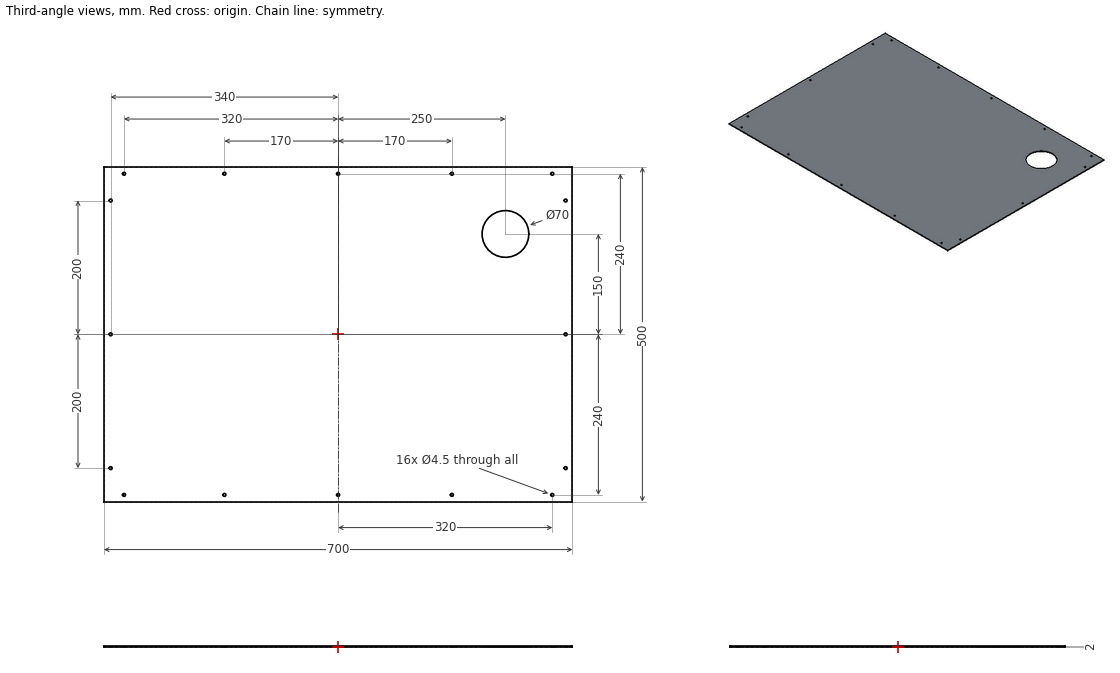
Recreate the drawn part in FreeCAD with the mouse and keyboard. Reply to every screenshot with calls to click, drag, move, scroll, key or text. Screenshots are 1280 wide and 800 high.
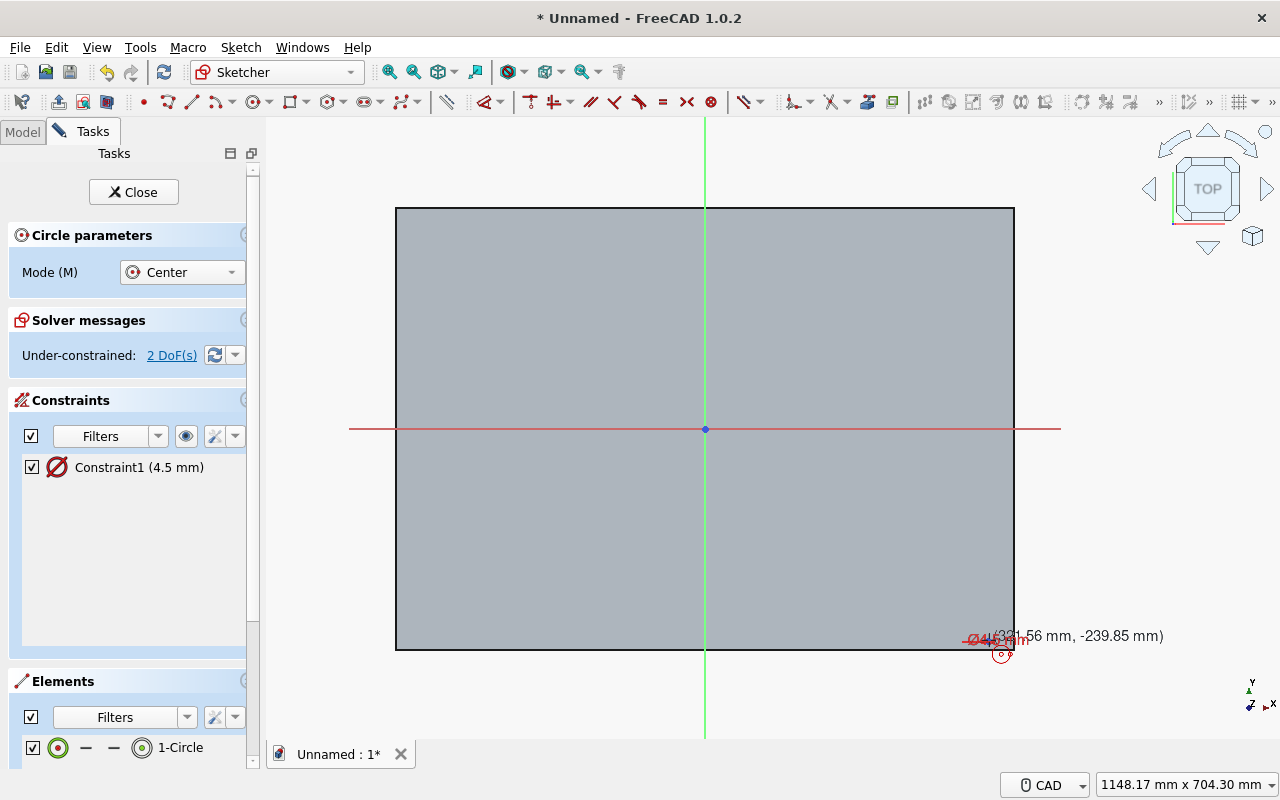
scroll(405, 429, up, 13)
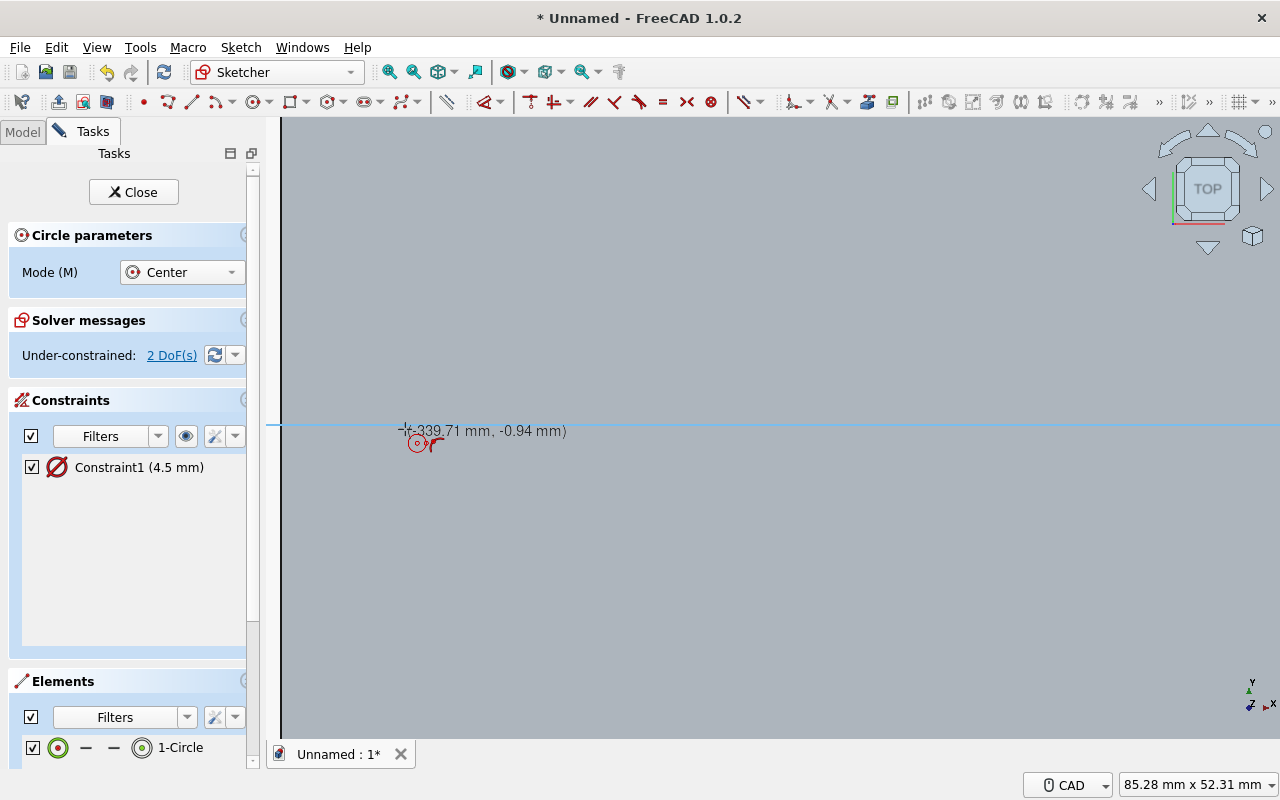
scroll(405, 428, down, 13)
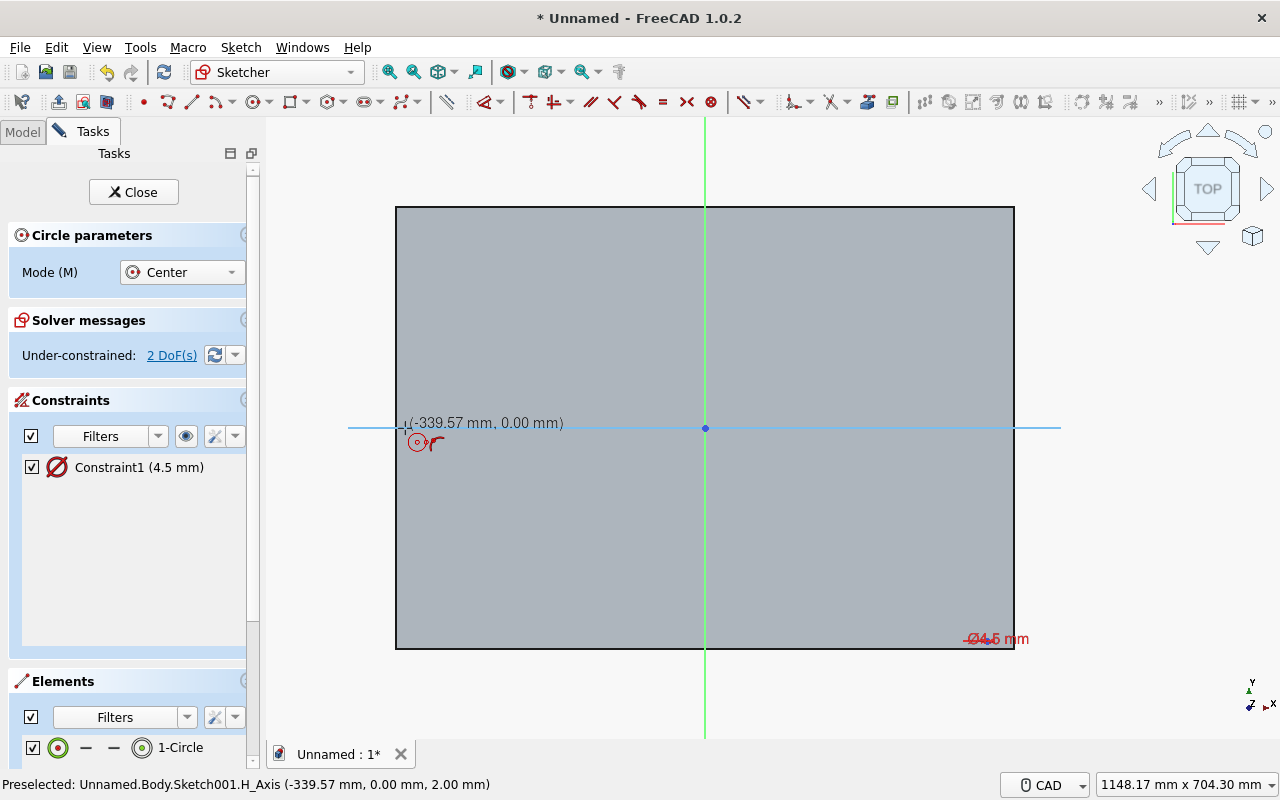
click(405, 428)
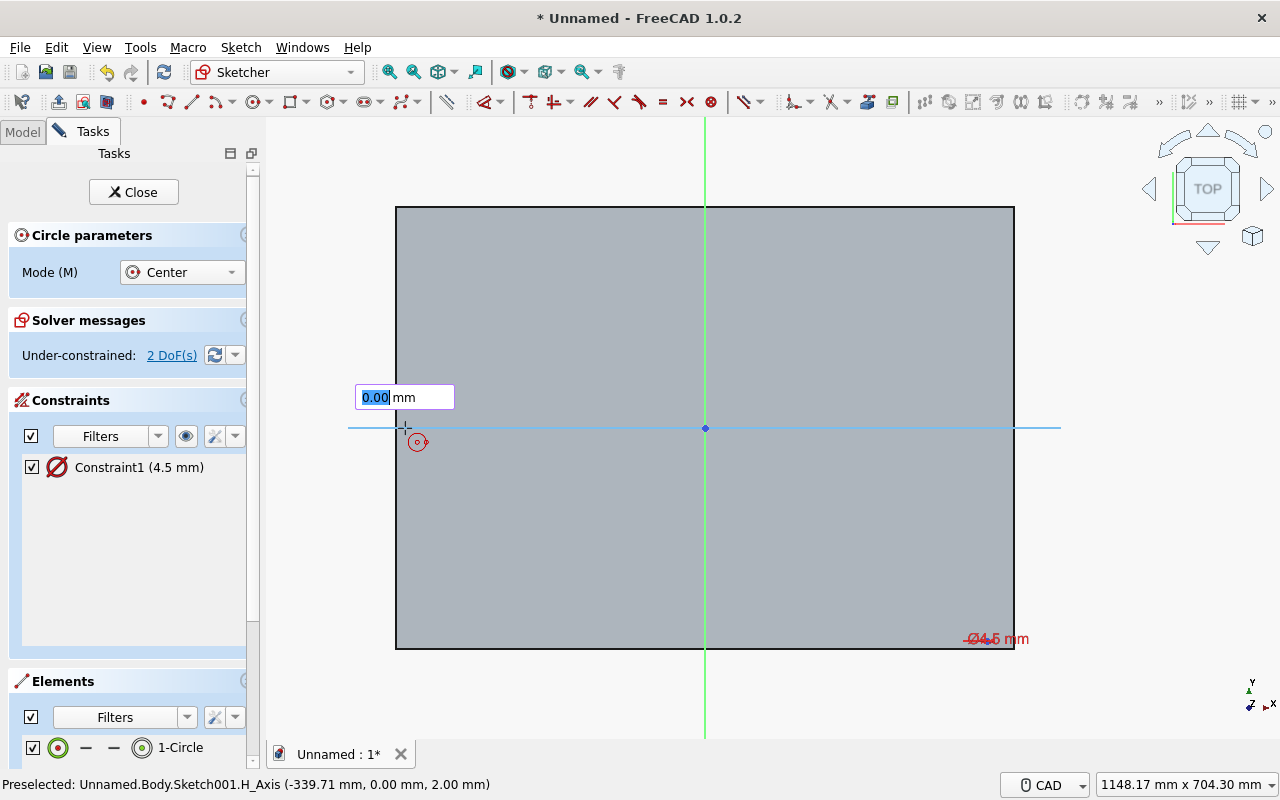
scroll(404, 430, up, 11)
move(404, 427)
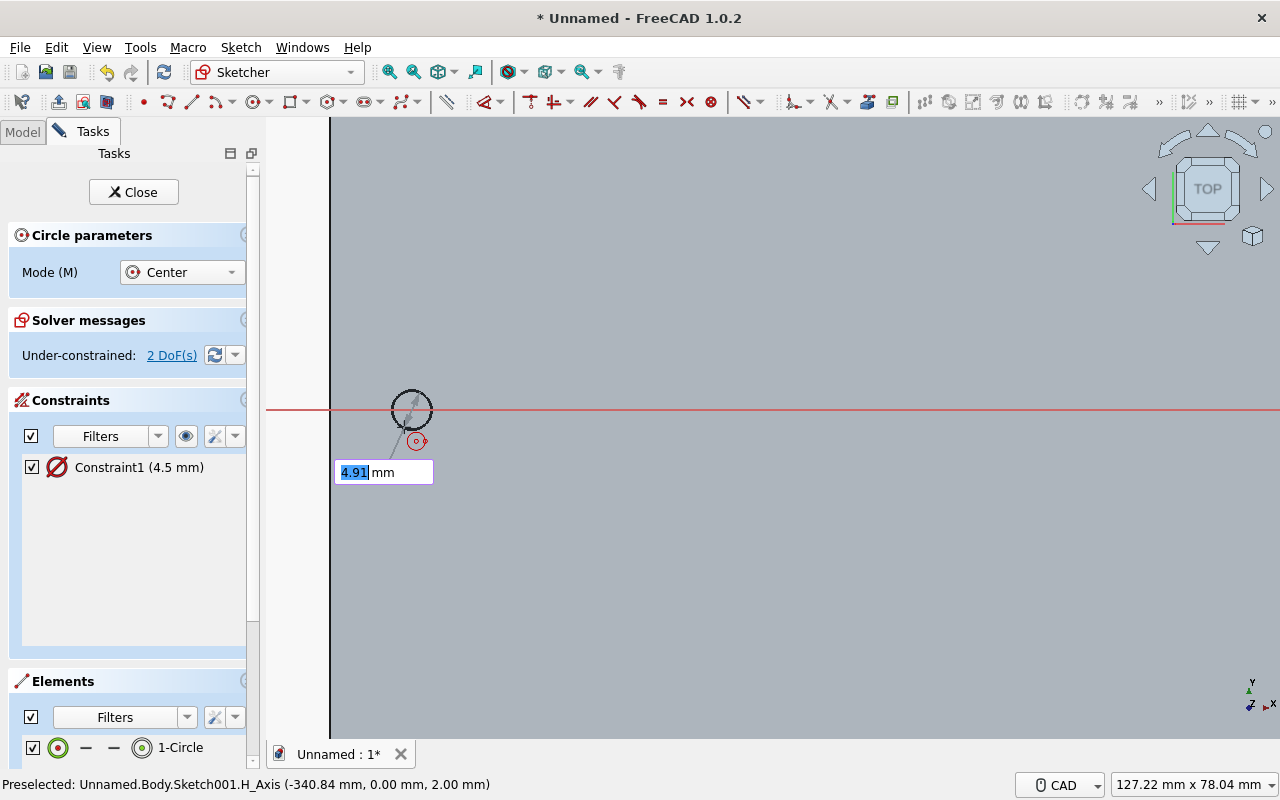
text(4.5)
key(Return)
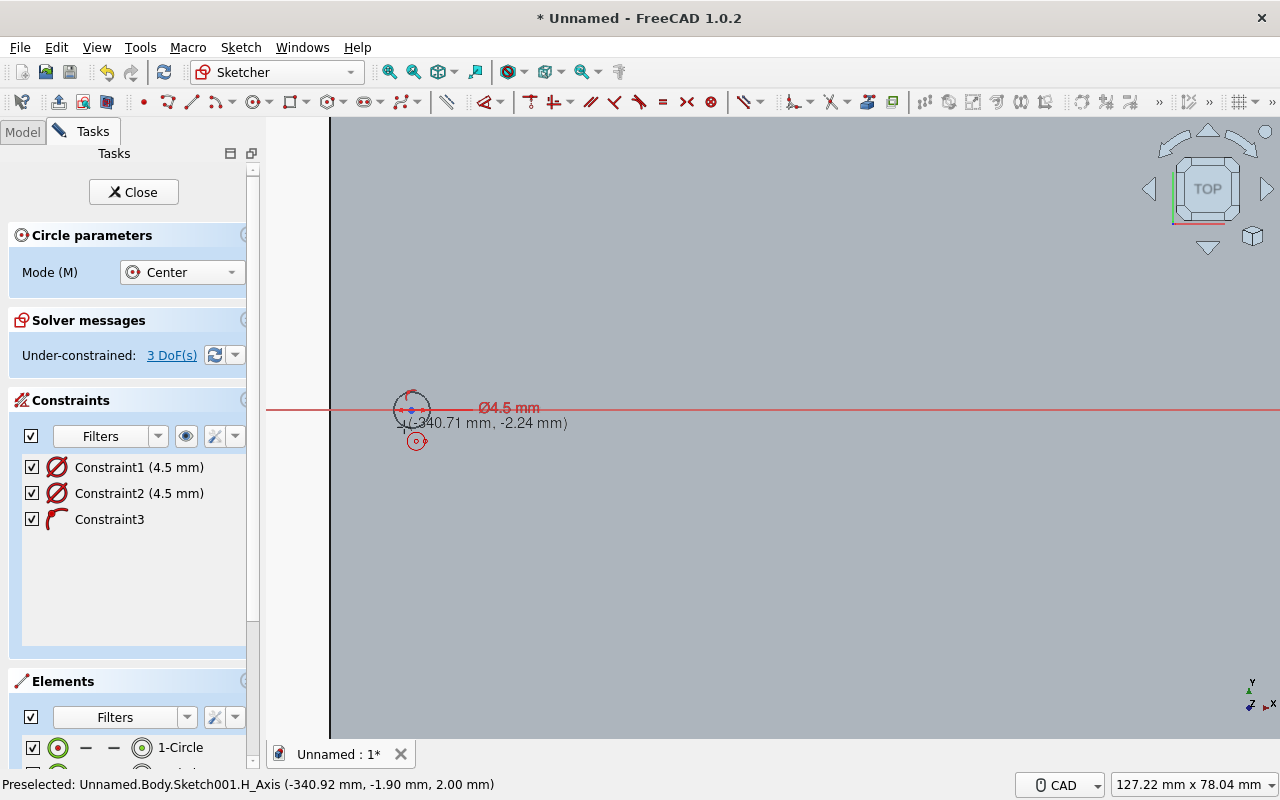
scroll(404, 430, down, 11)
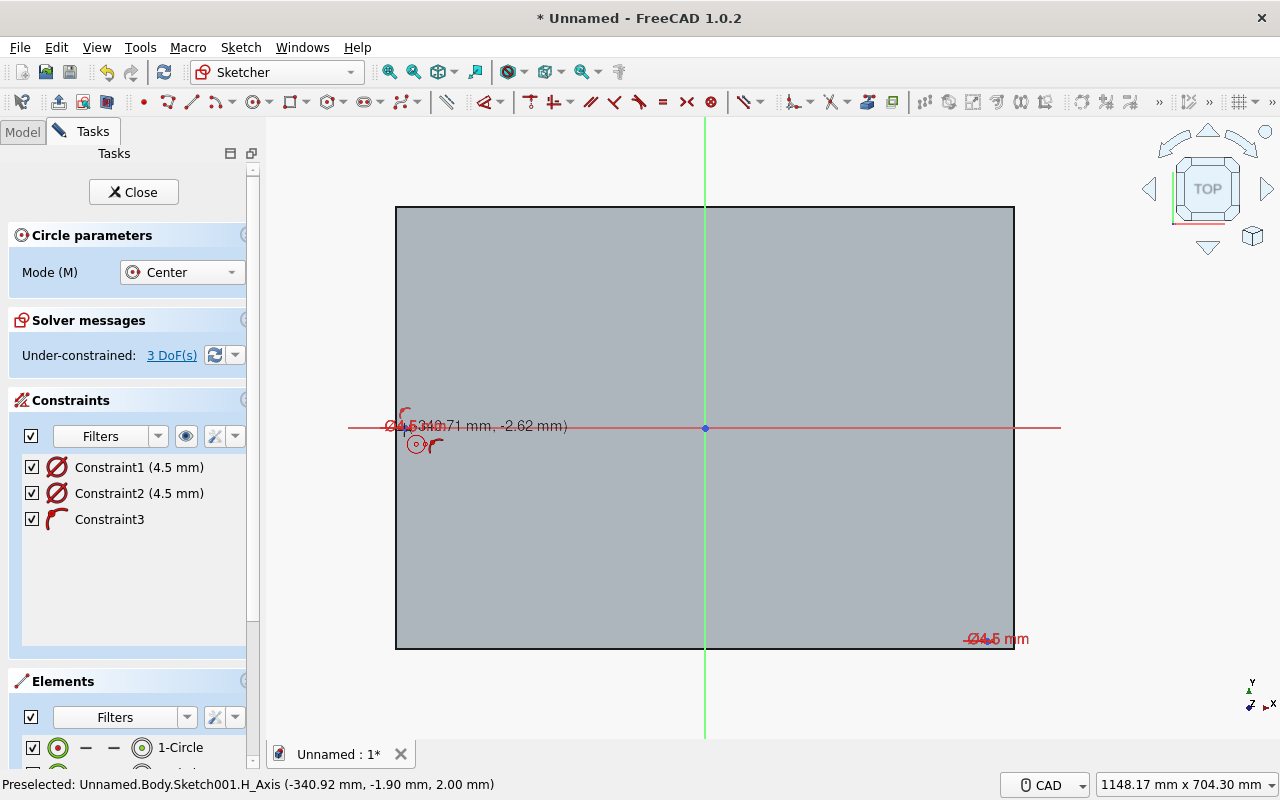
scroll(705, 640, up, 13)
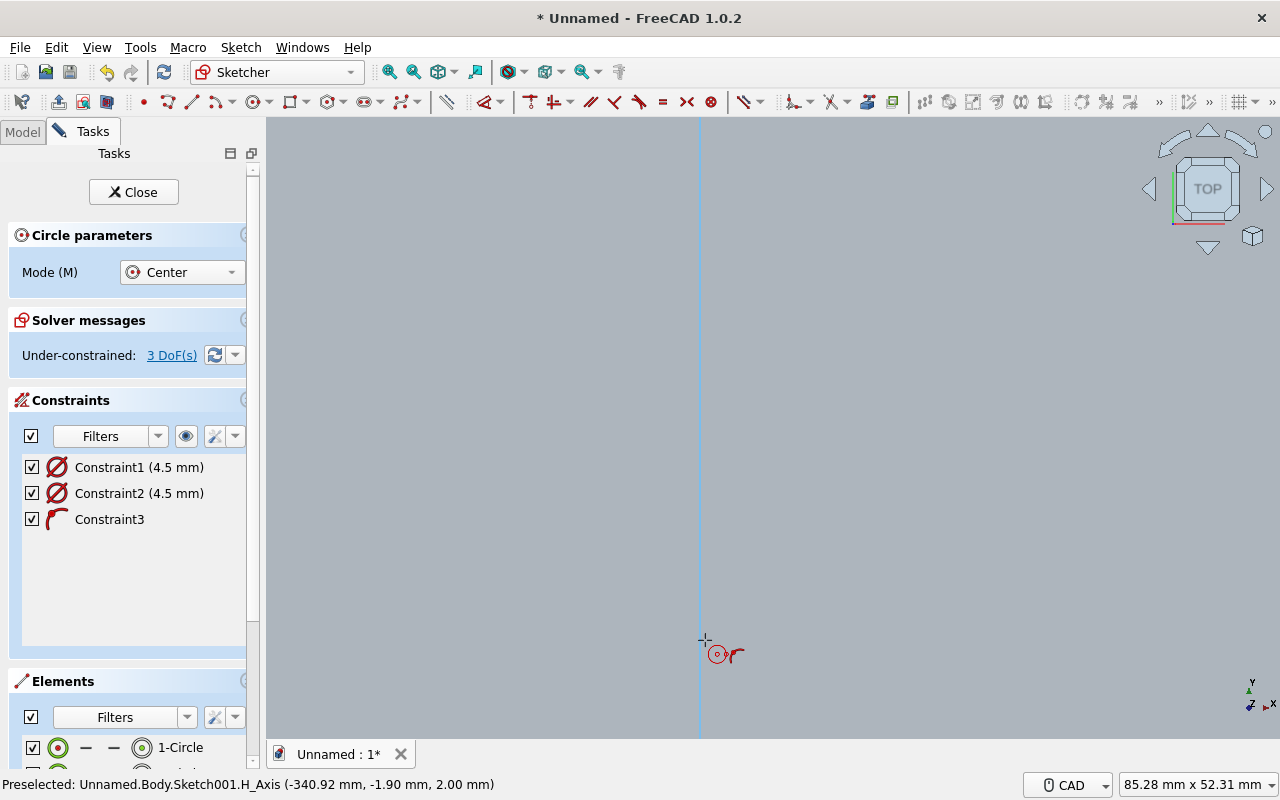
scroll(705, 641, down, 13)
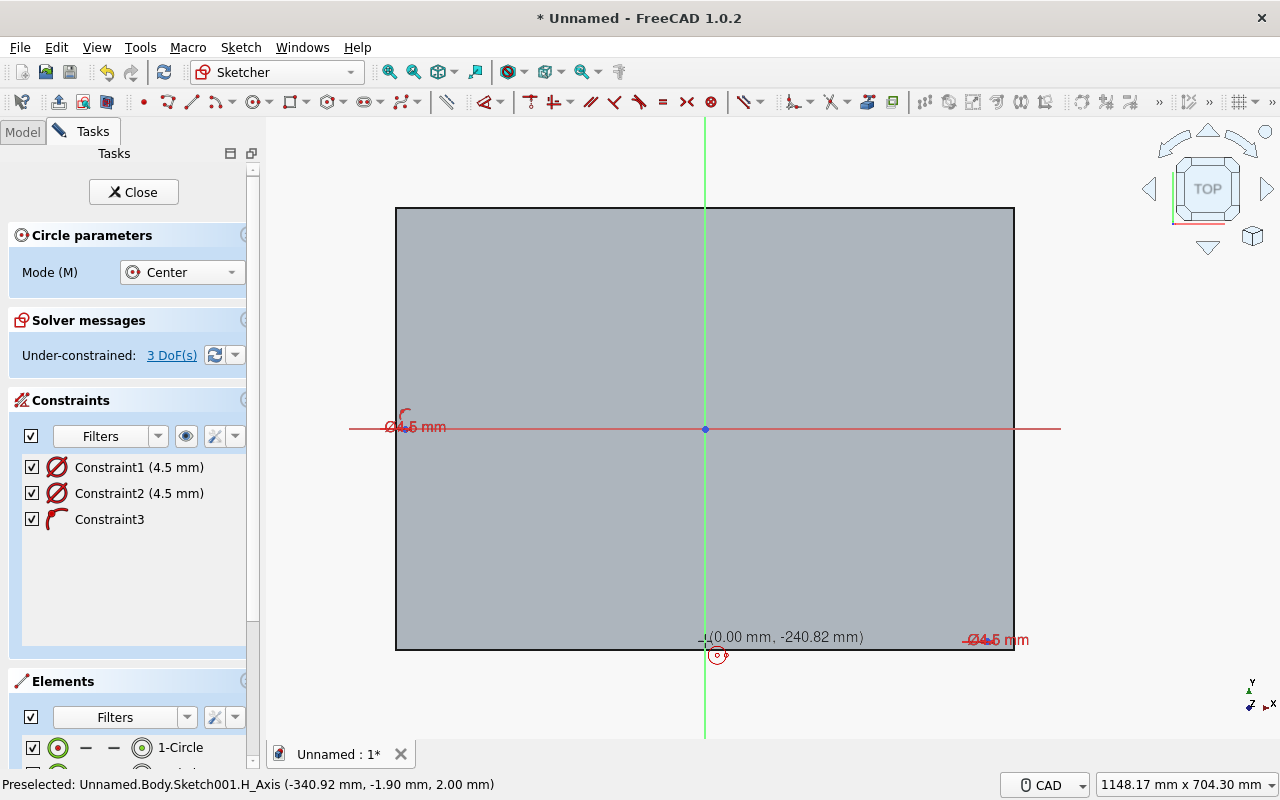
click(705, 641)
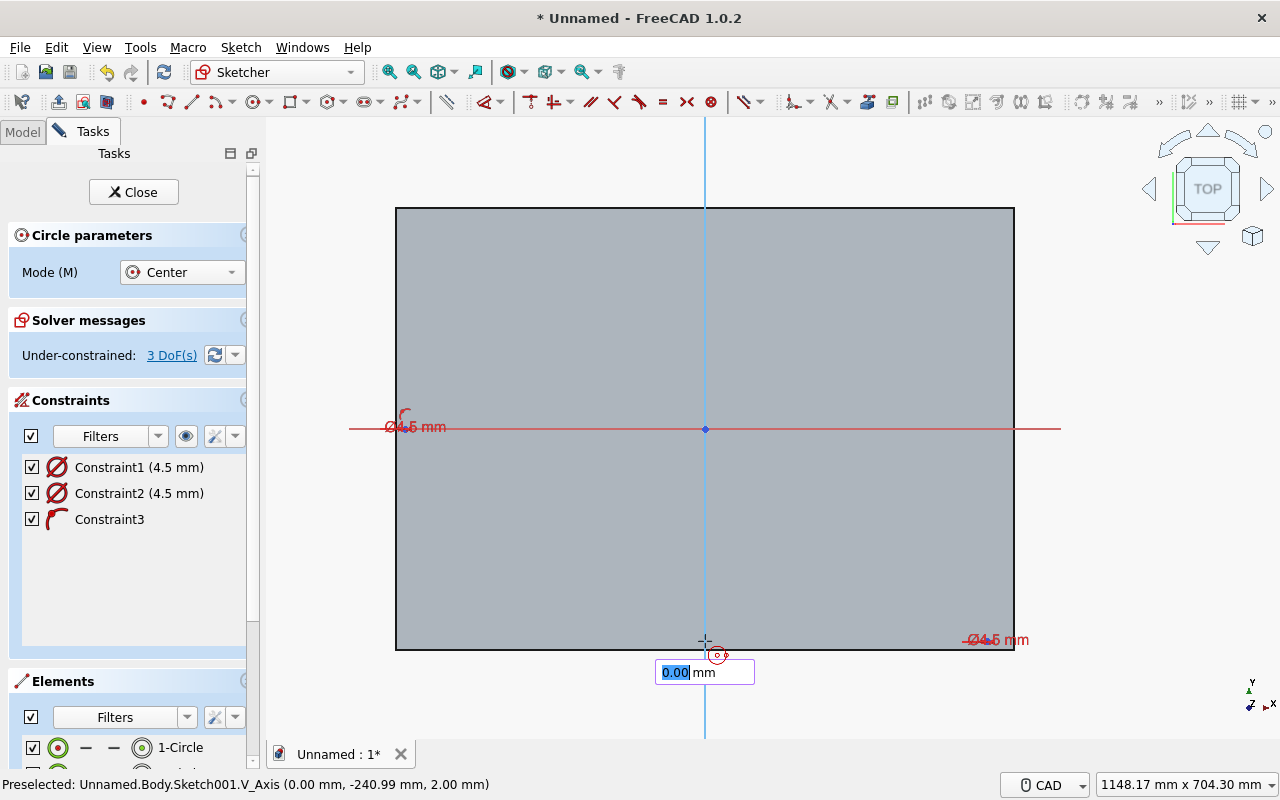
scroll(707, 640, up, 11)
move(702, 637)